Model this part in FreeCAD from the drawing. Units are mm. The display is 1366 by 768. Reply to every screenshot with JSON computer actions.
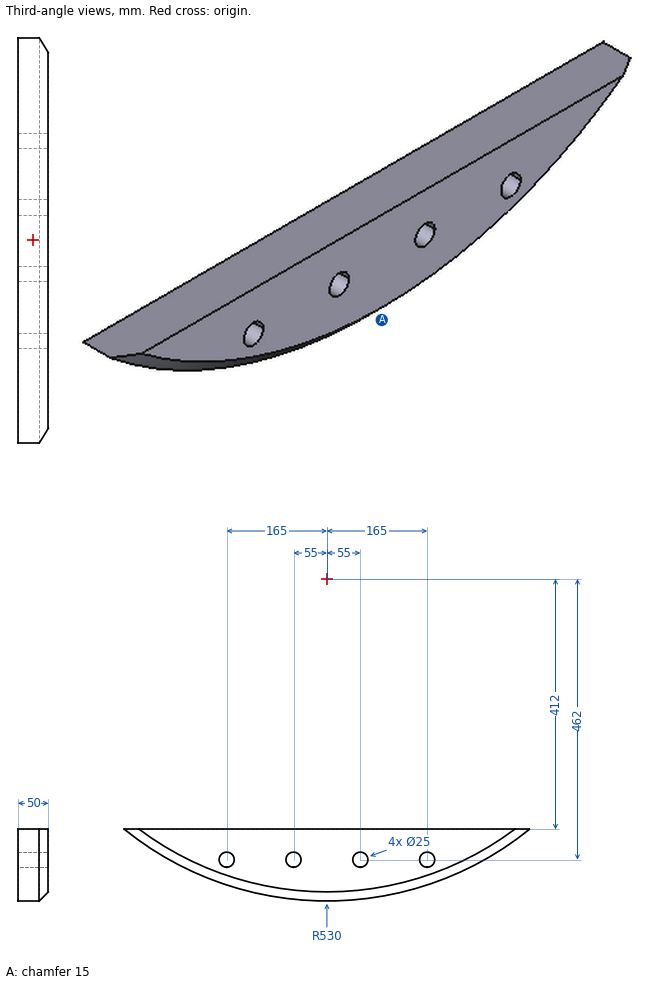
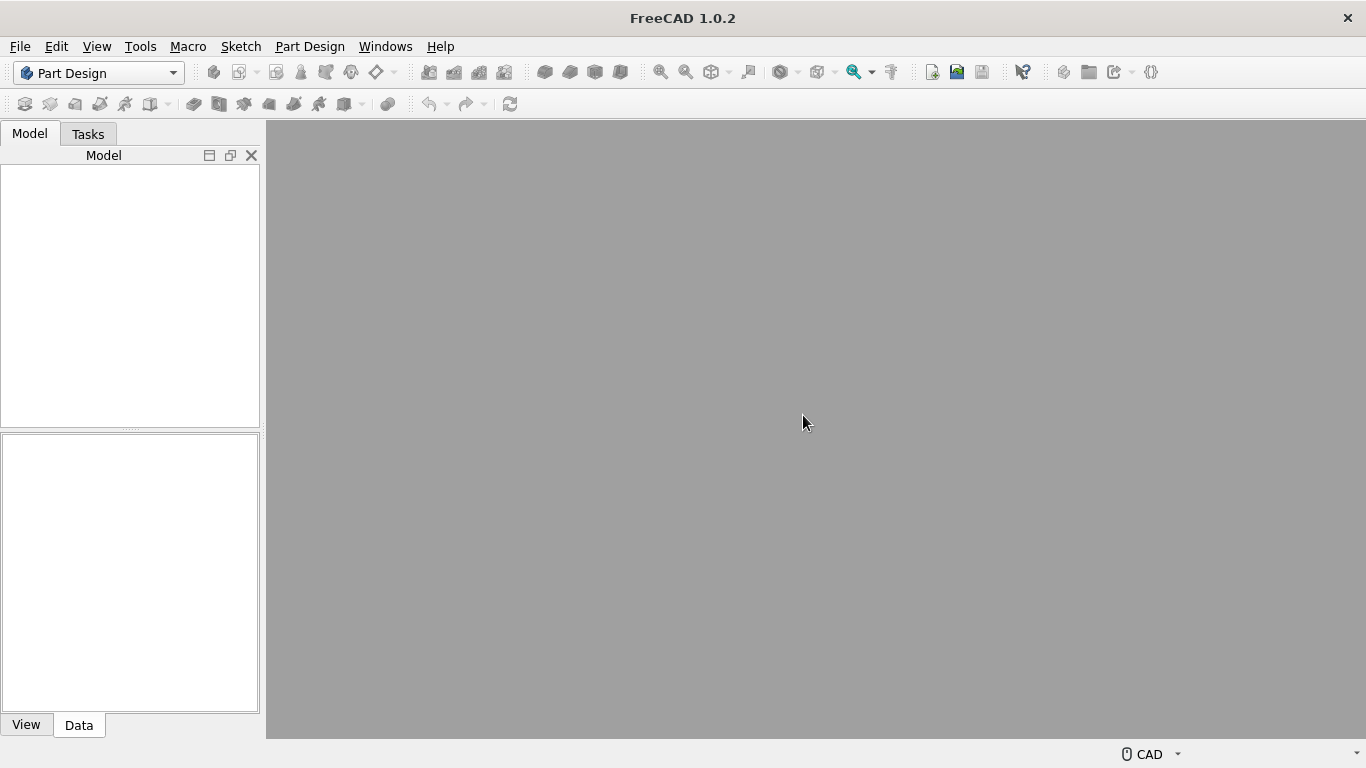
{"action": "left_click", "coordinate": [932, 72]}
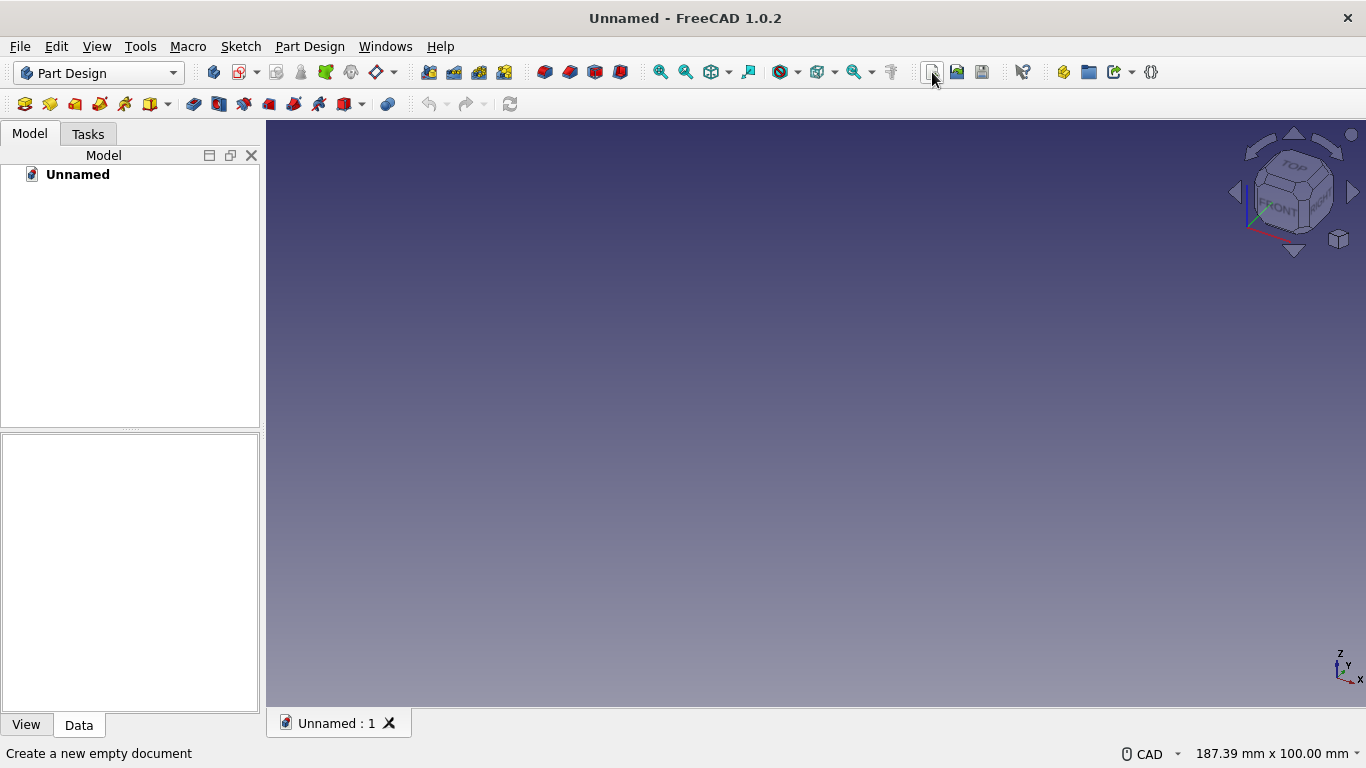
{"action": "left_click", "coordinate": [238, 72]}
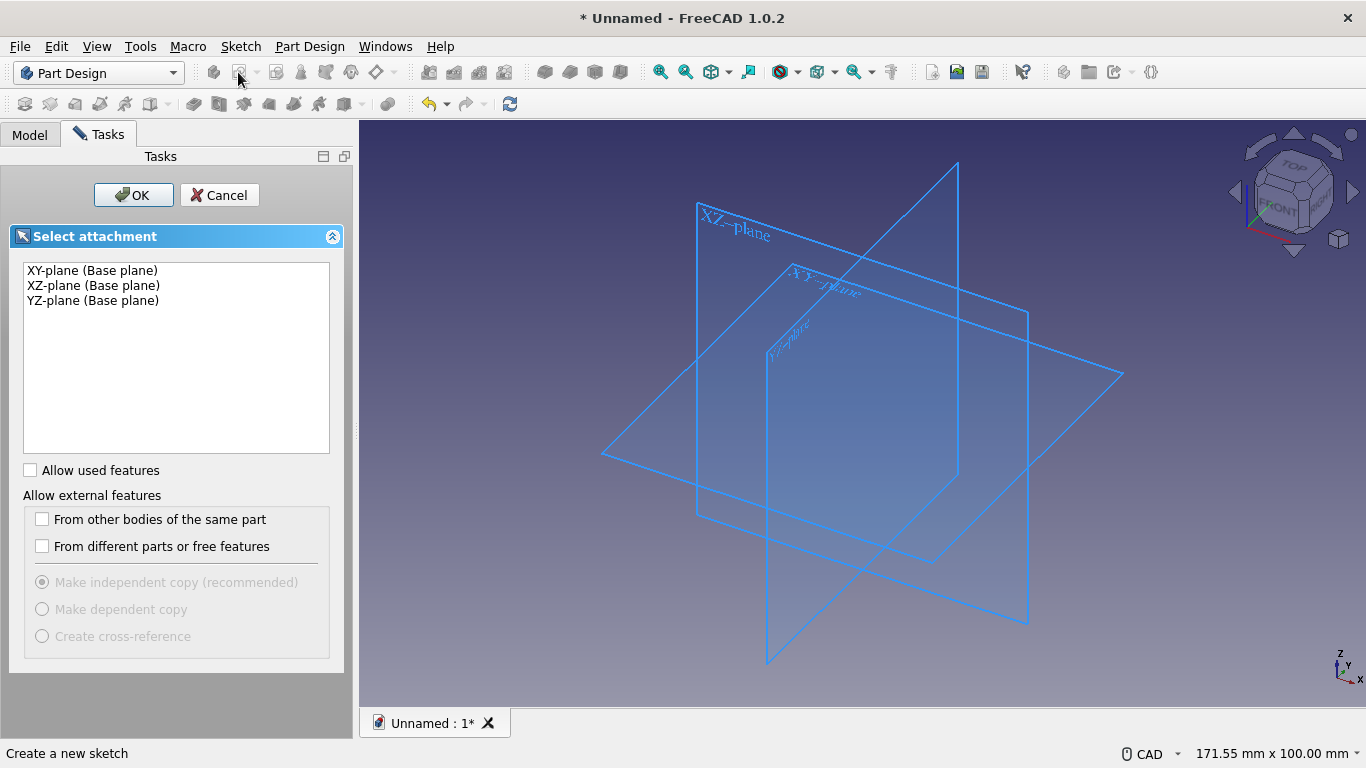
{"action": "left_click", "coordinate": [84, 300]}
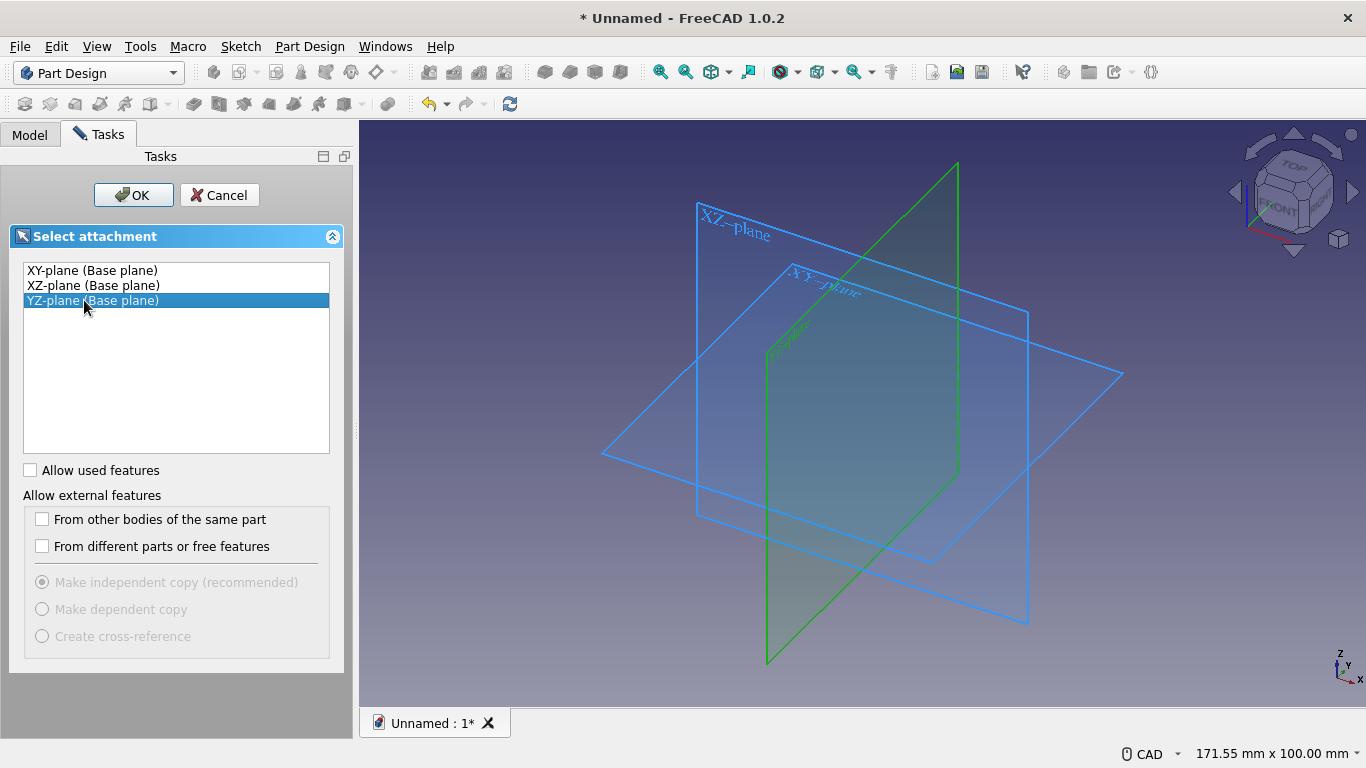
{"action": "left_click", "coordinate": [134, 195]}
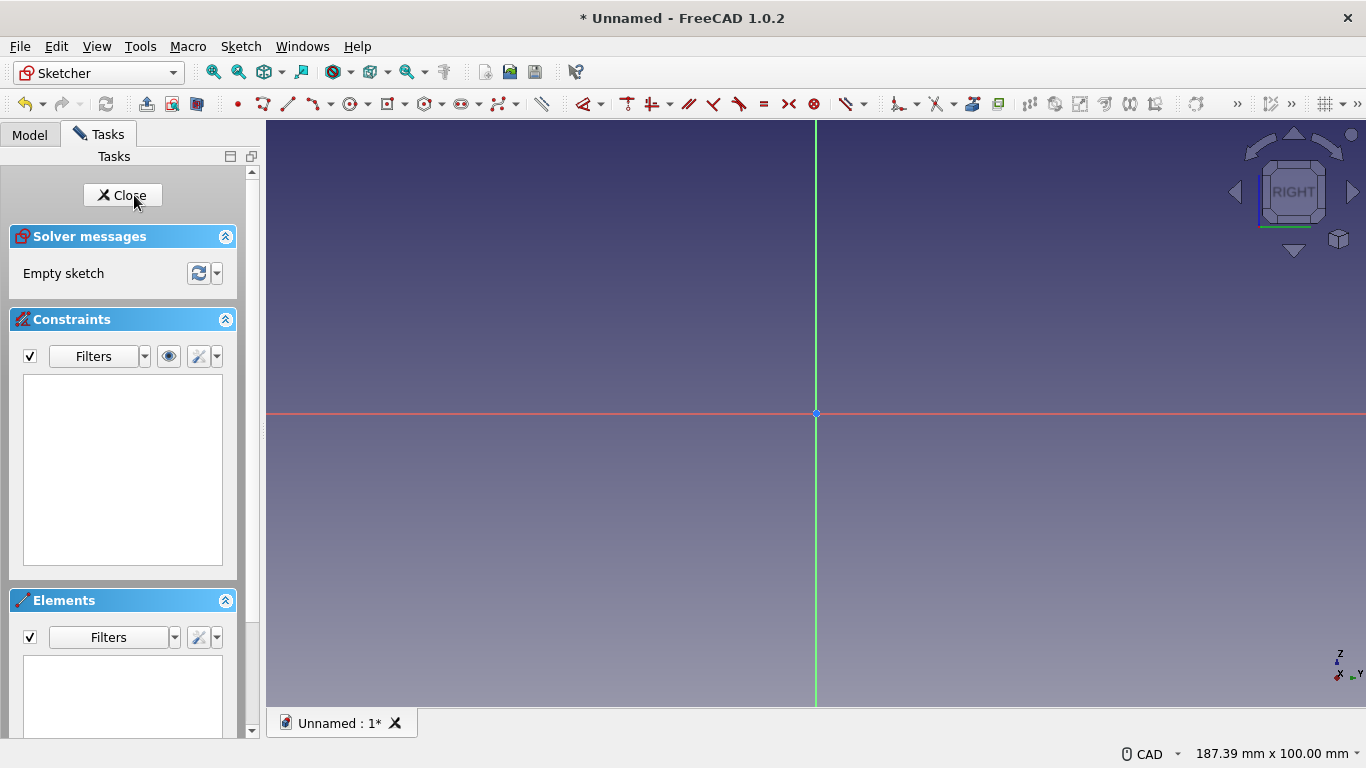
{"action": "scroll", "coordinate": [739, 220], "scroll_direction": "down", "scroll_amount": 11}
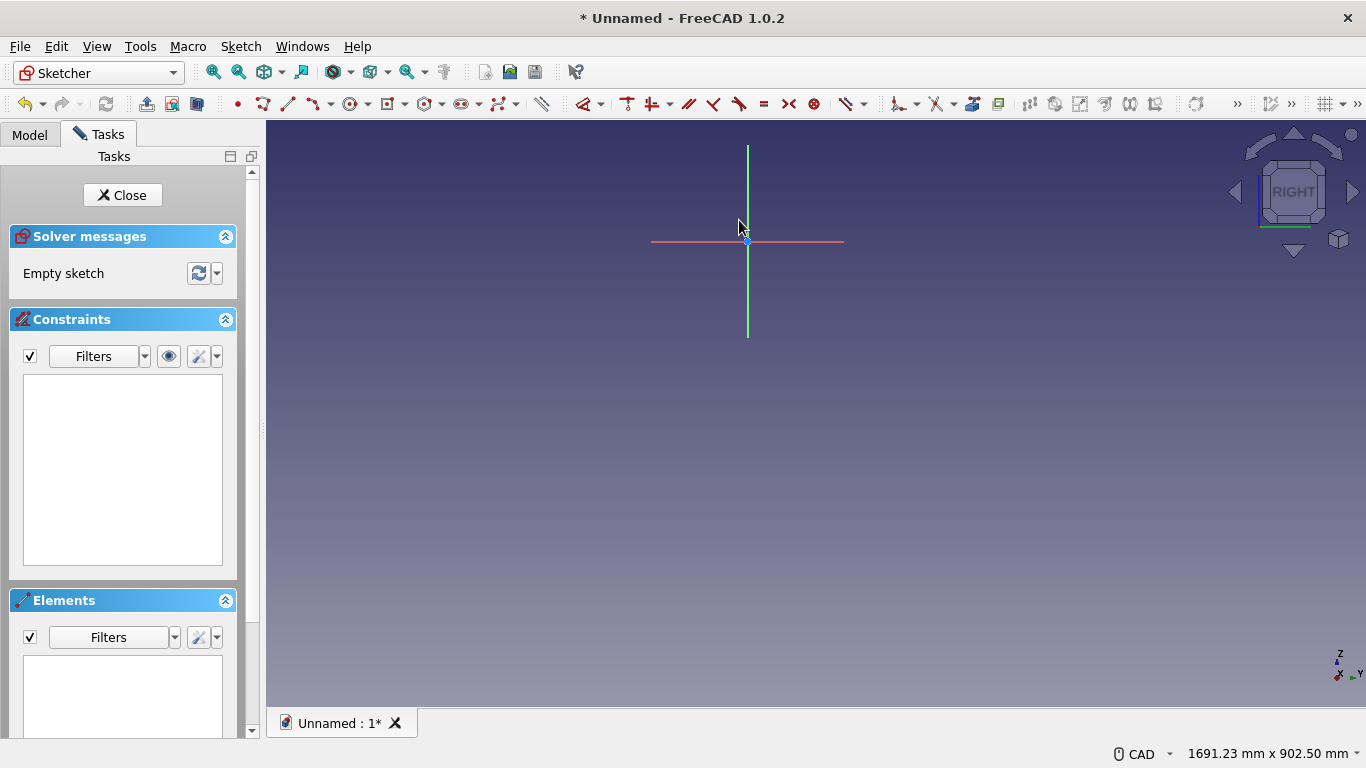
{"action": "left_click", "coordinate": [288, 104]}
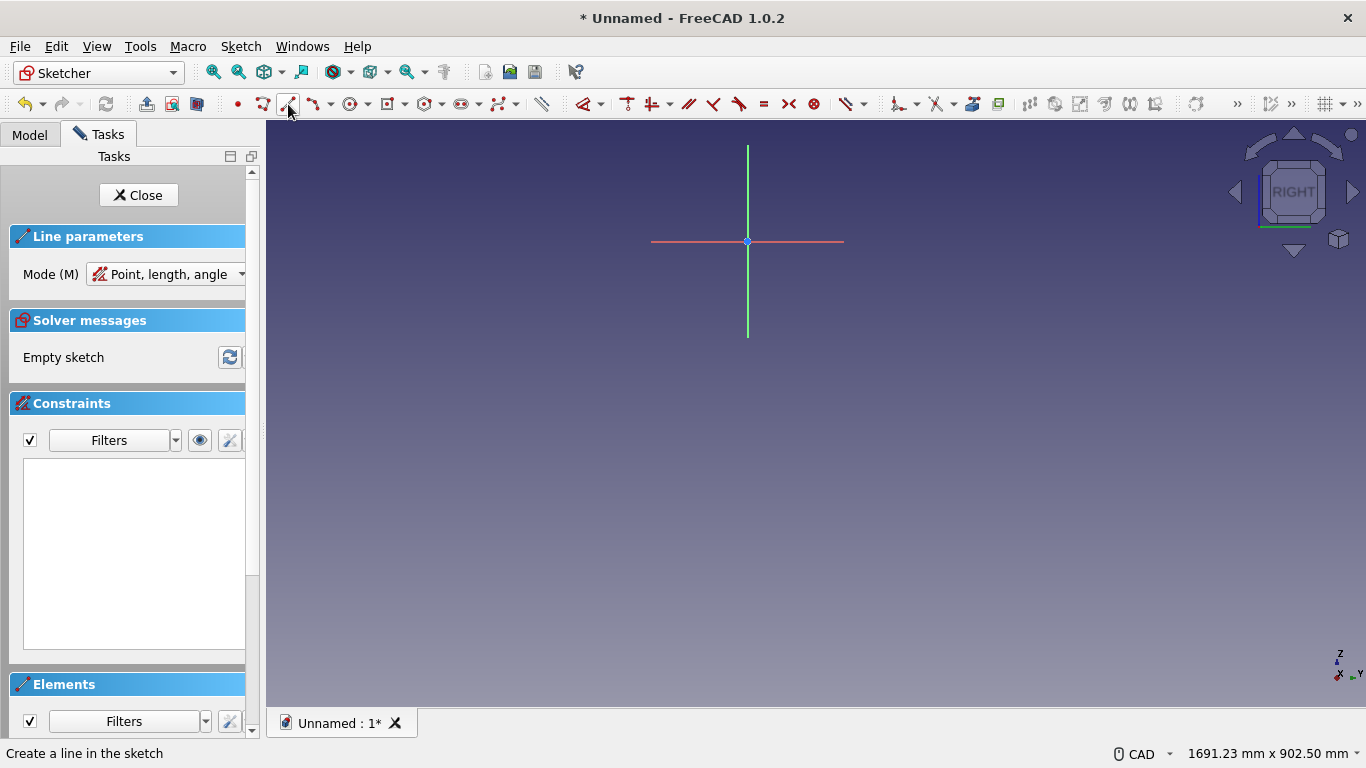
{"action": "left_click", "coordinate": [965, 510]}
{"action": "left_click", "coordinate": [531, 510]}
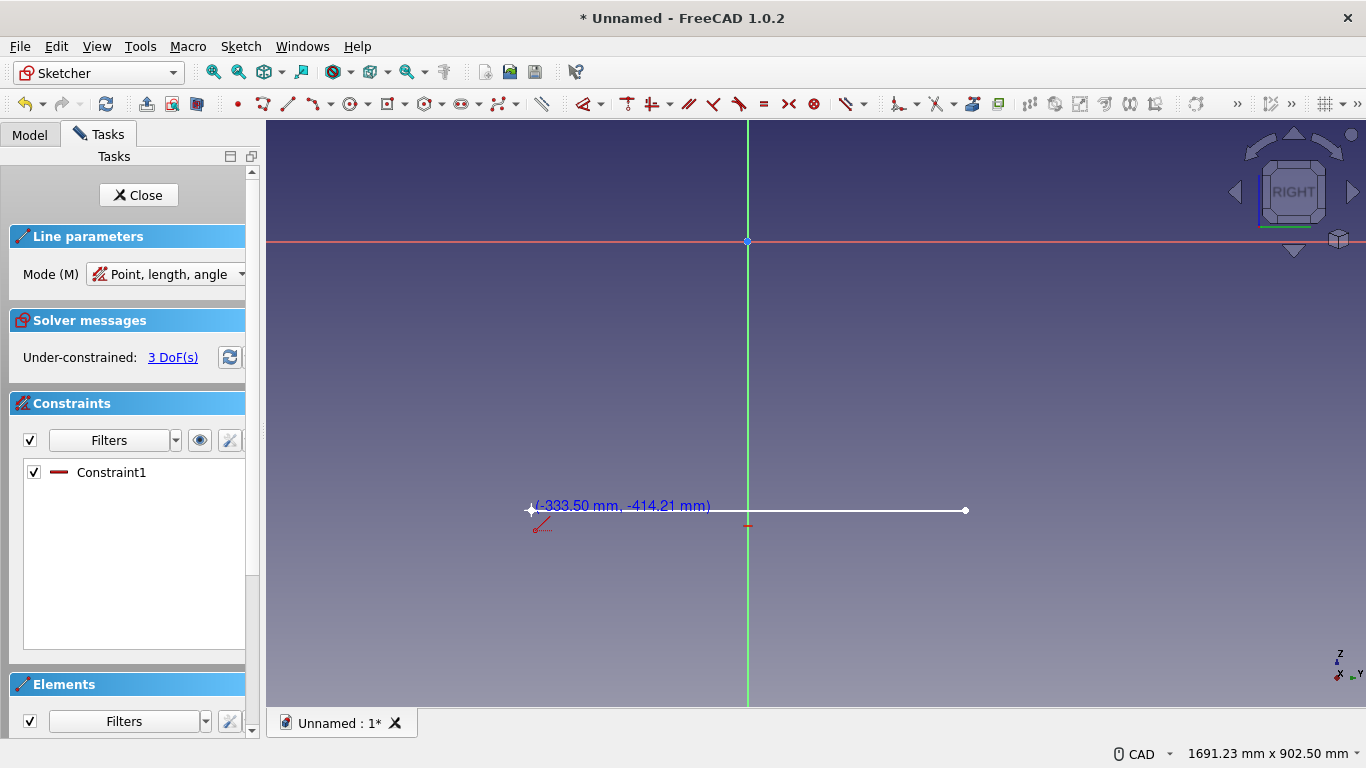
{"action": "left_click", "coordinate": [312, 104]}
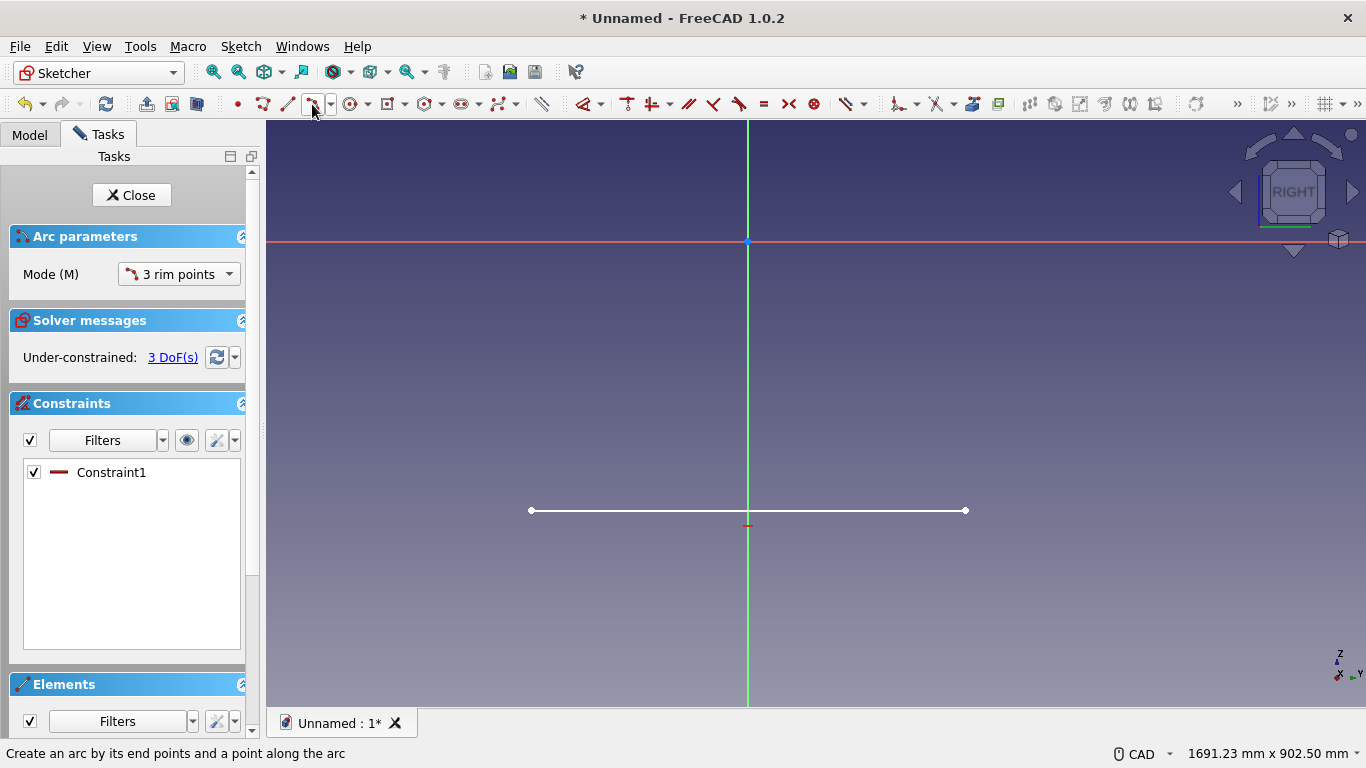
{"action": "left_click", "coordinate": [531, 511]}
{"action": "left_click", "coordinate": [965, 511]}
{"action": "left_click", "coordinate": [701, 583]}
{"action": "key", "text": "Escape"}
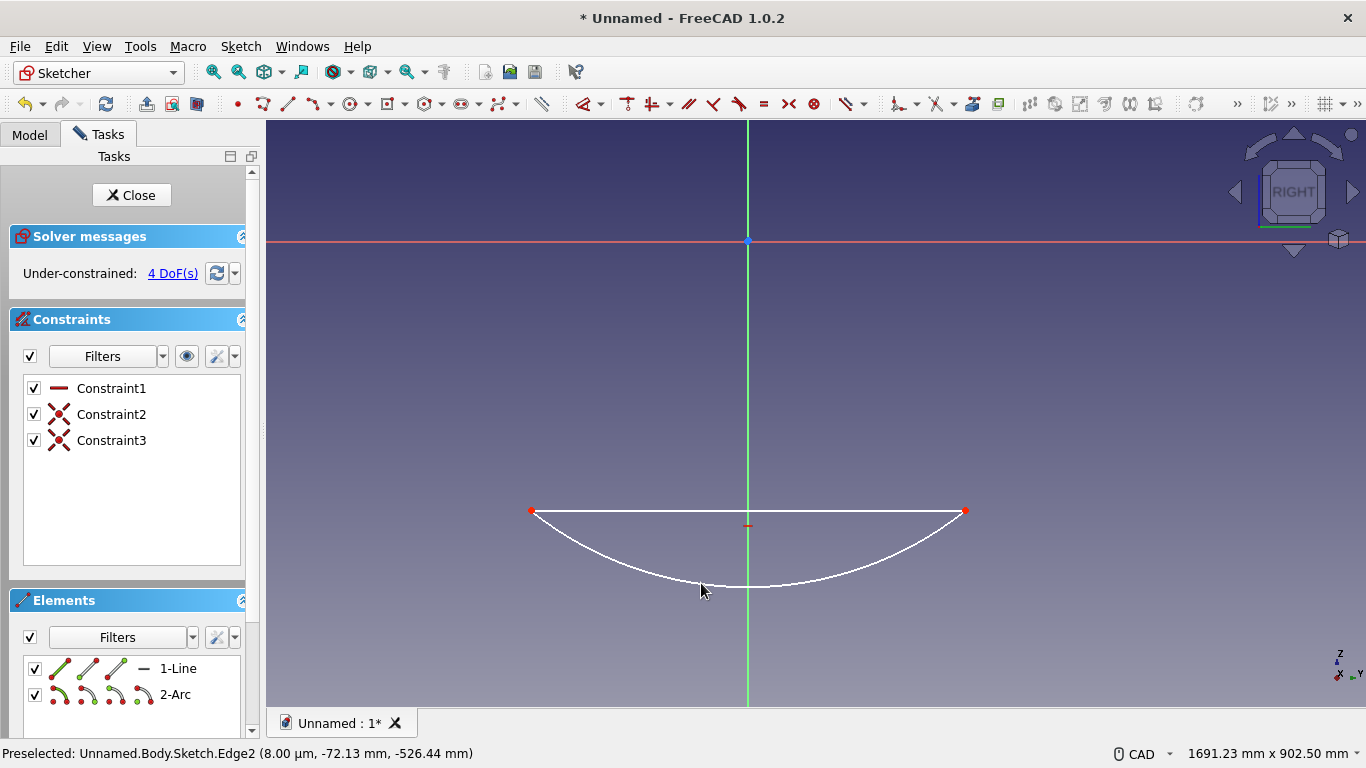
{"action": "left_click_drag", "start_coordinate": [738, 230], "coordinate": [758, 252]}